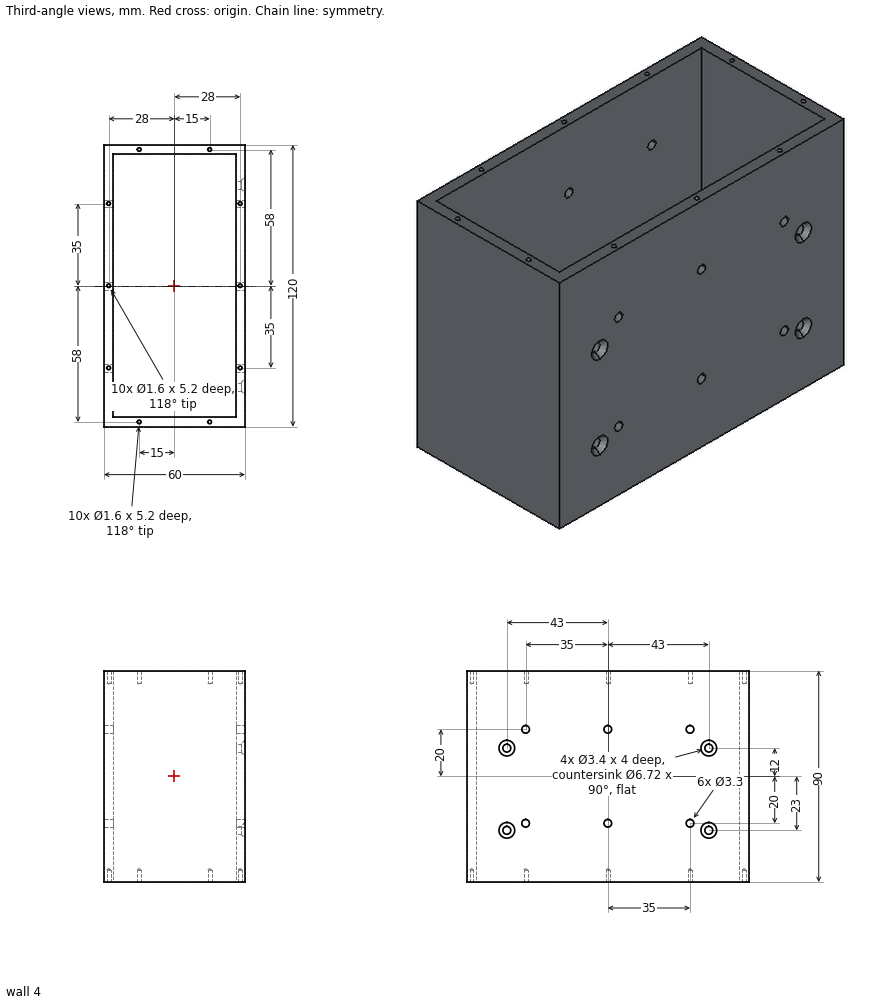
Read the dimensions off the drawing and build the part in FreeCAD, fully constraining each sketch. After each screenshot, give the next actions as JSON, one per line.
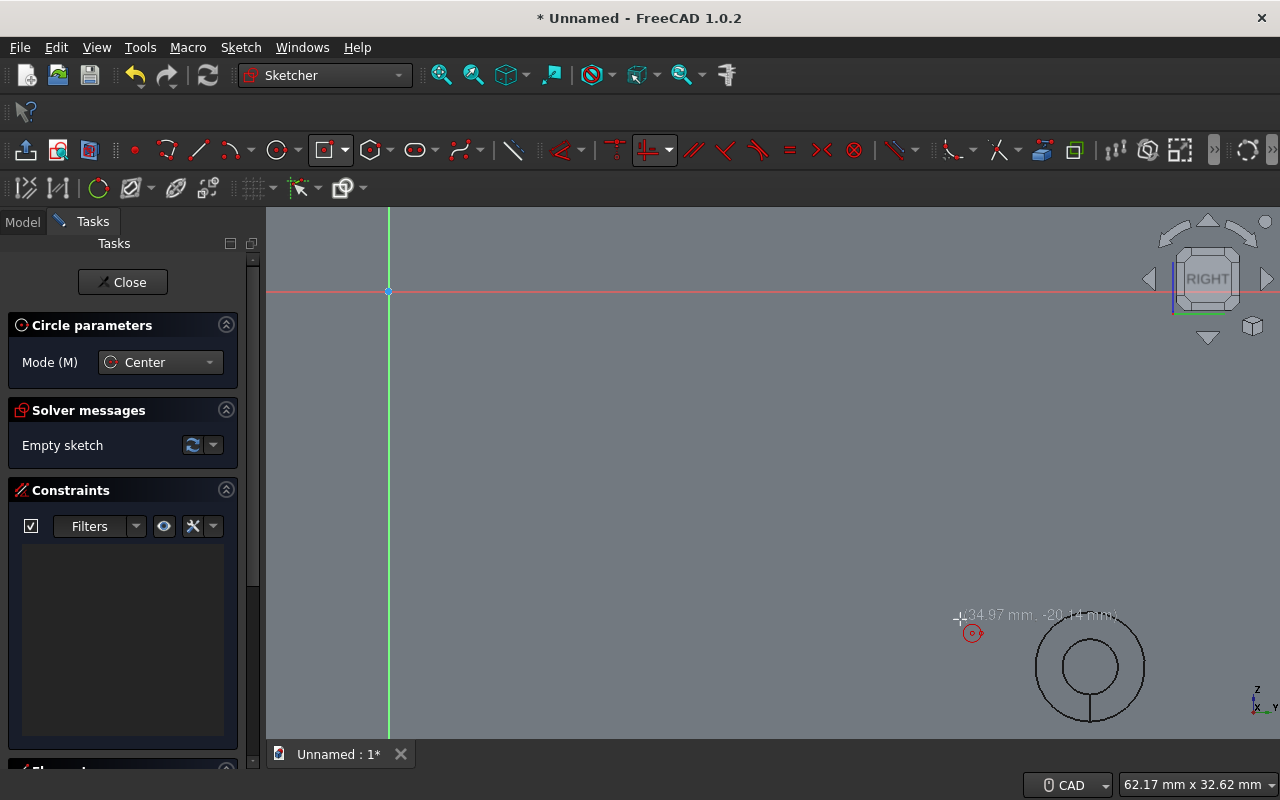
{"action": "left_click", "coordinate": [960, 618]}
{"action": "mouse_move", "coordinate": [979, 599]}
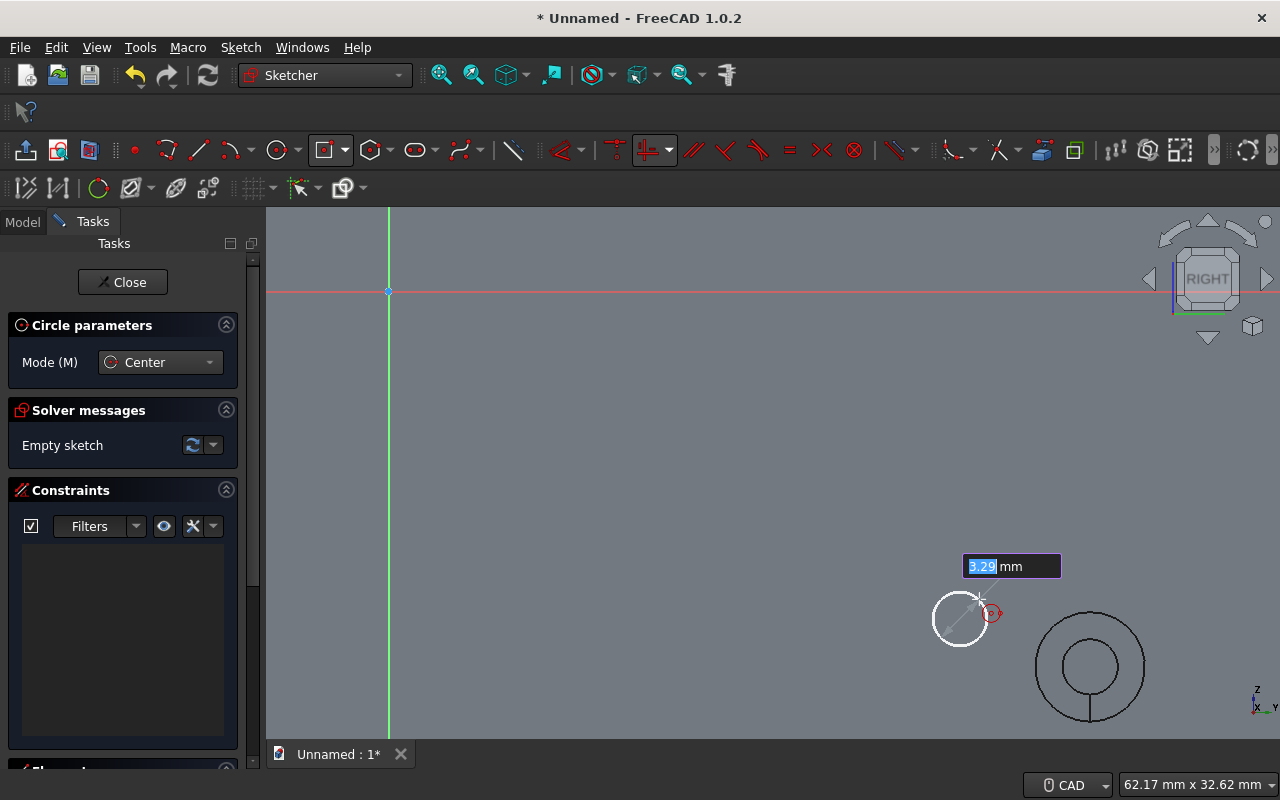
{"action": "type", "text": "3.3"}
{"action": "key", "text": "Return"}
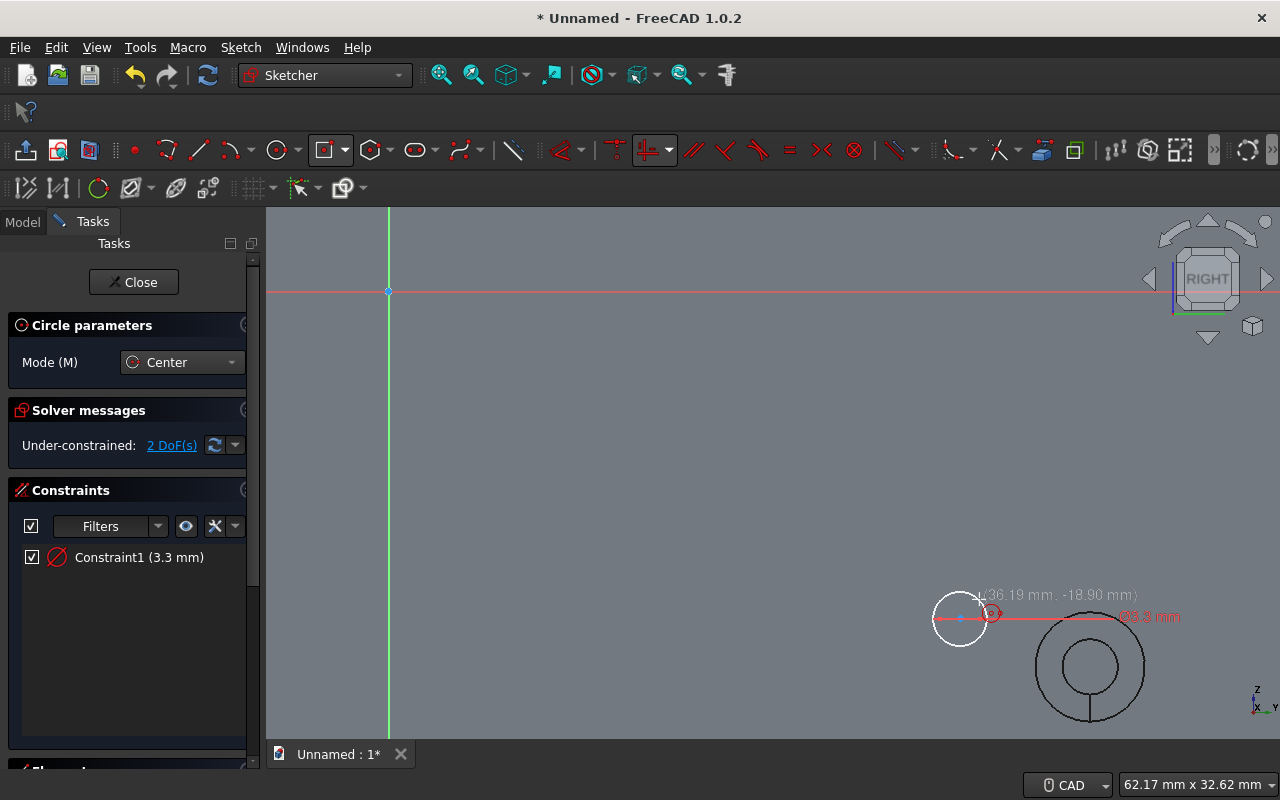
{"action": "scroll", "coordinate": [962, 621], "scroll_direction": "down", "scroll_amount": 4}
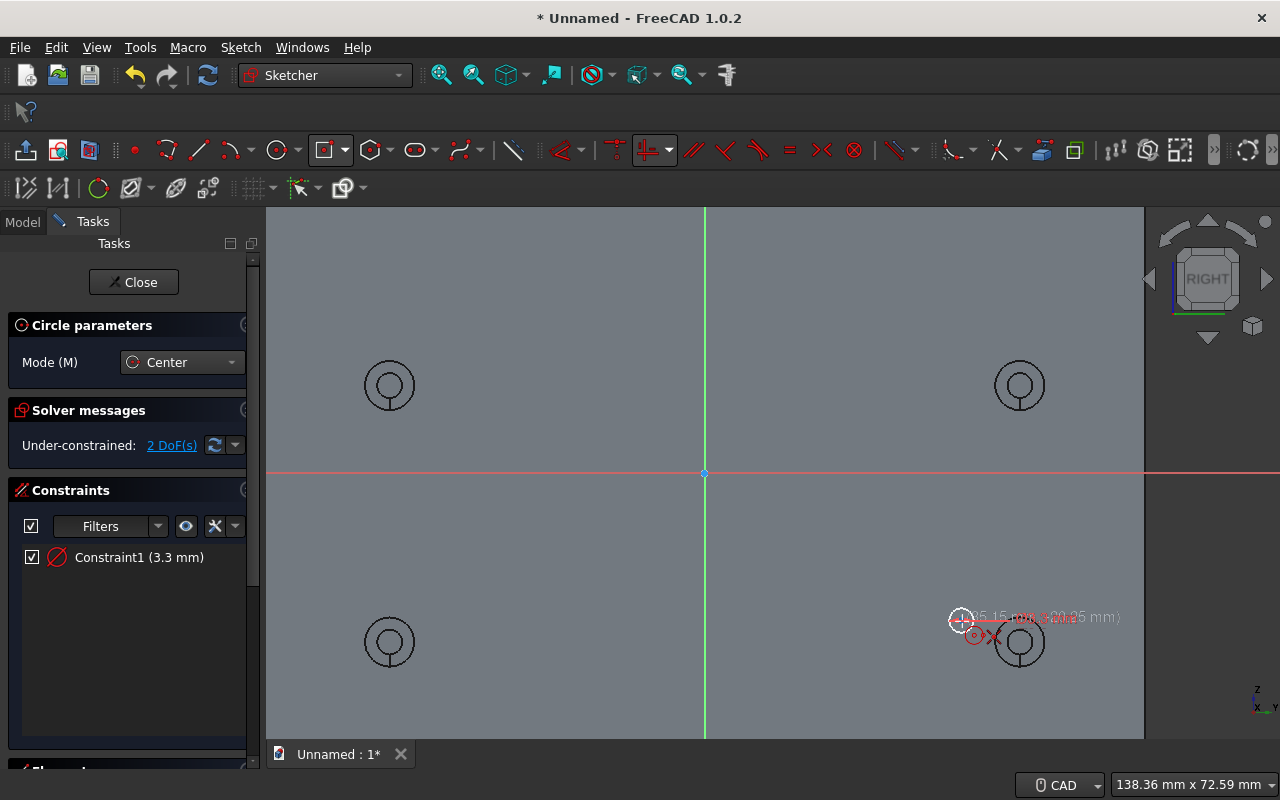
{"action": "scroll", "coordinate": [448, 327], "scroll_direction": "up", "scroll_amount": 4}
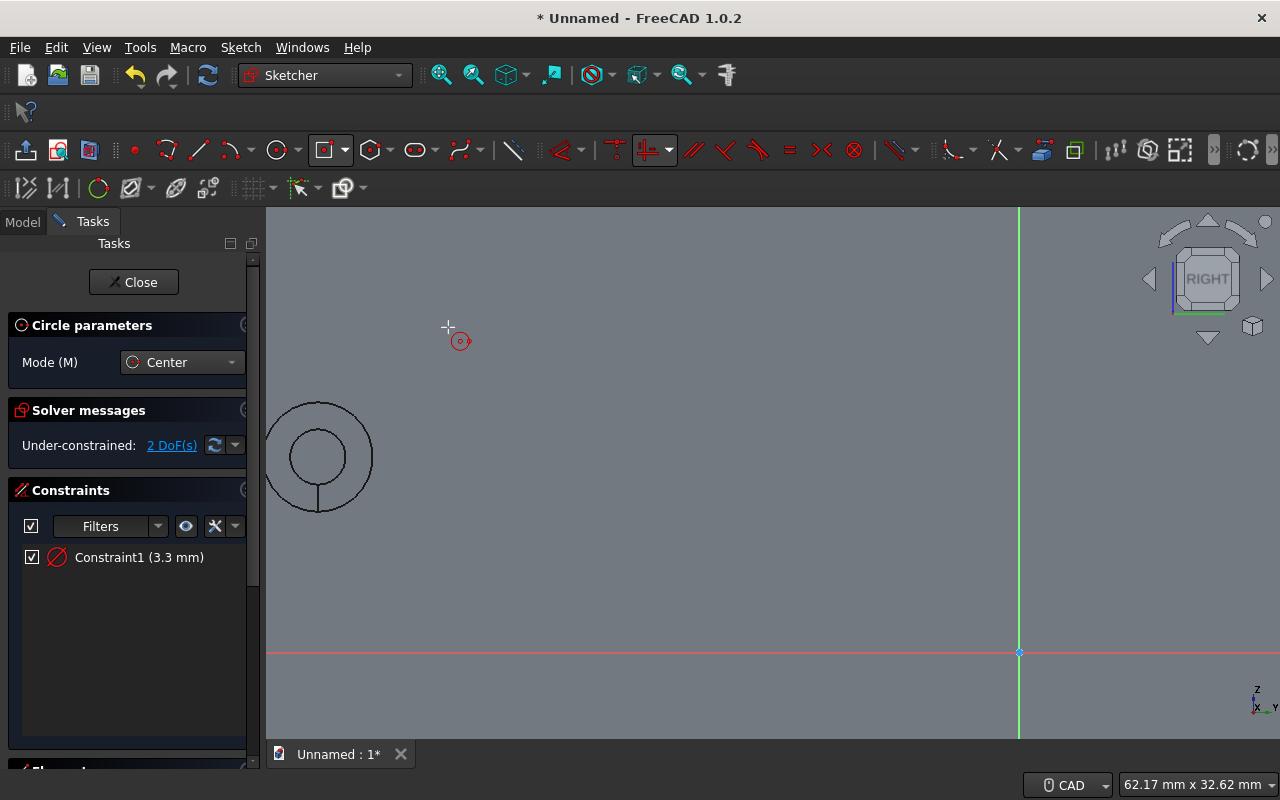
{"action": "left_click", "coordinate": [448, 327]}
{"action": "mouse_move", "coordinate": [467, 308]}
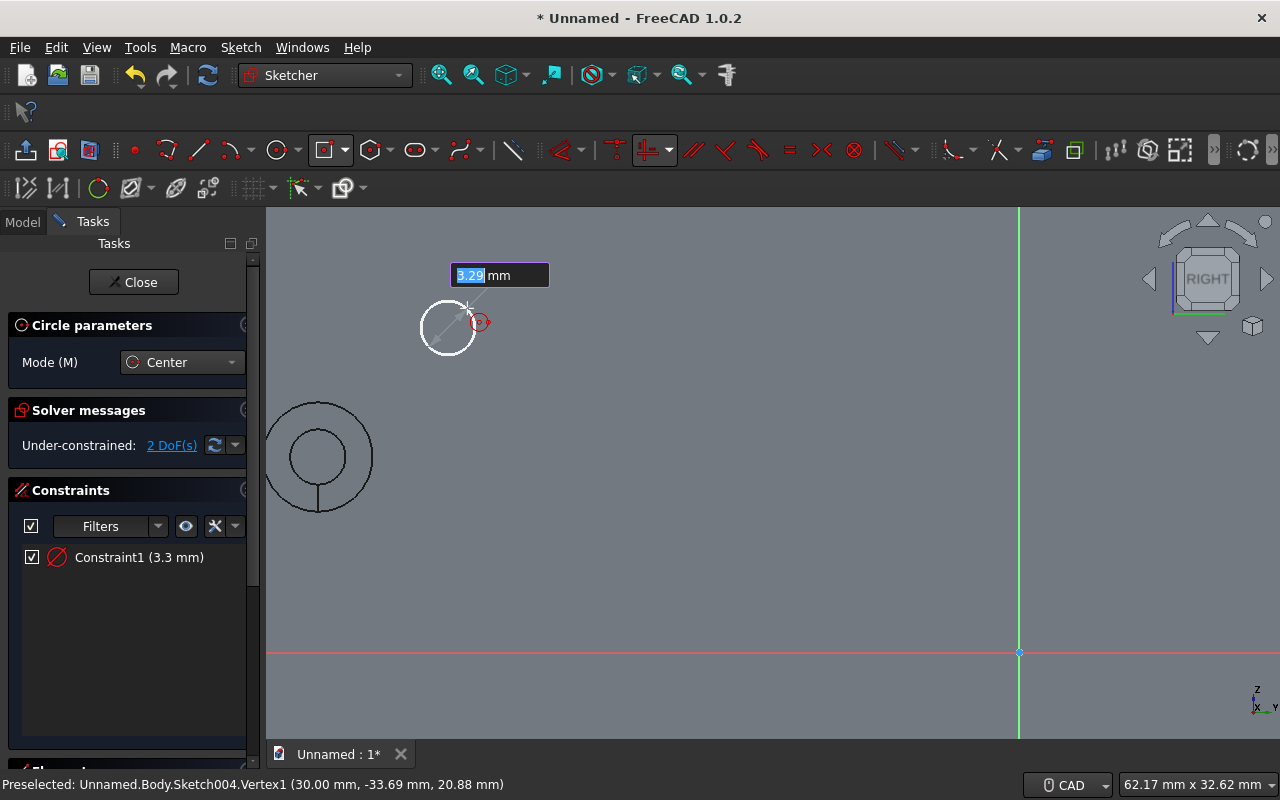
{"action": "type", "text": "3.3"}
{"action": "key", "text": "Return"}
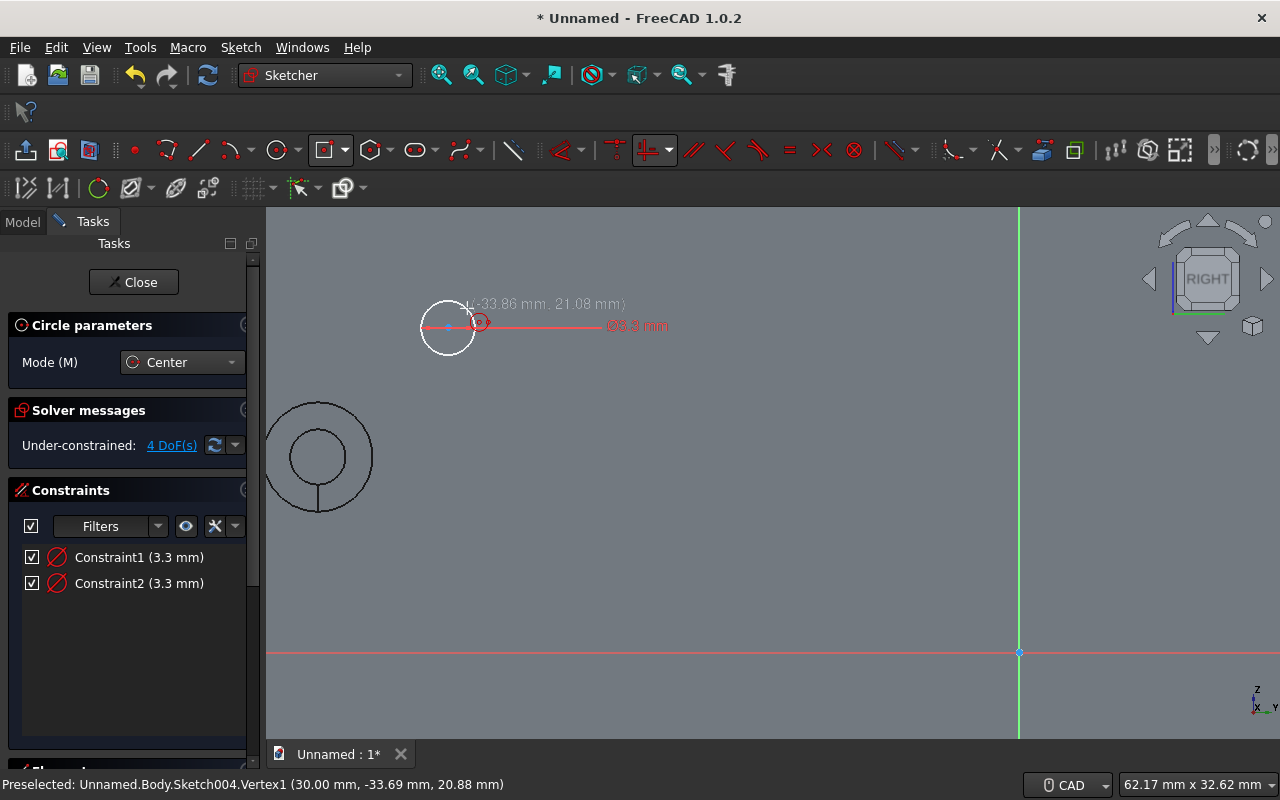
{"action": "scroll", "coordinate": [448, 326], "scroll_direction": "down", "scroll_amount": 4}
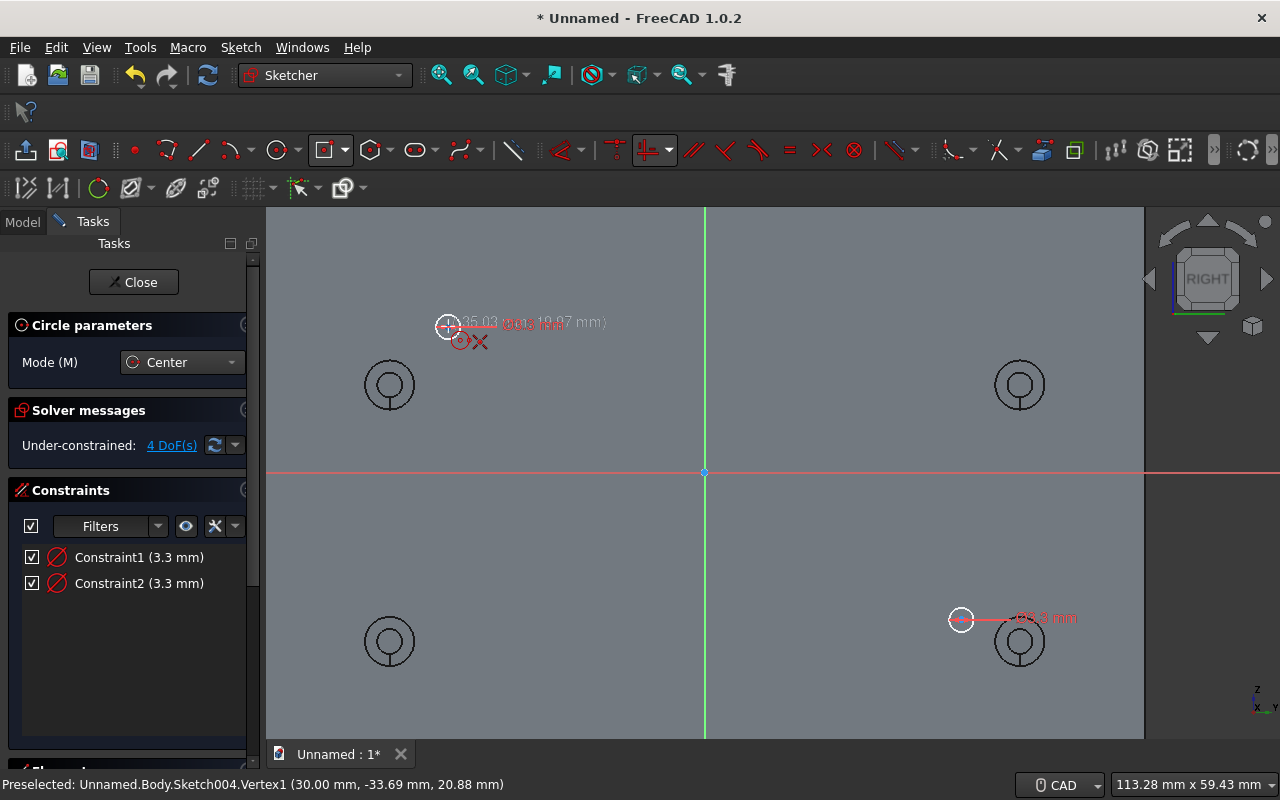
{"action": "scroll", "coordinate": [961, 326], "scroll_direction": "up", "scroll_amount": 4}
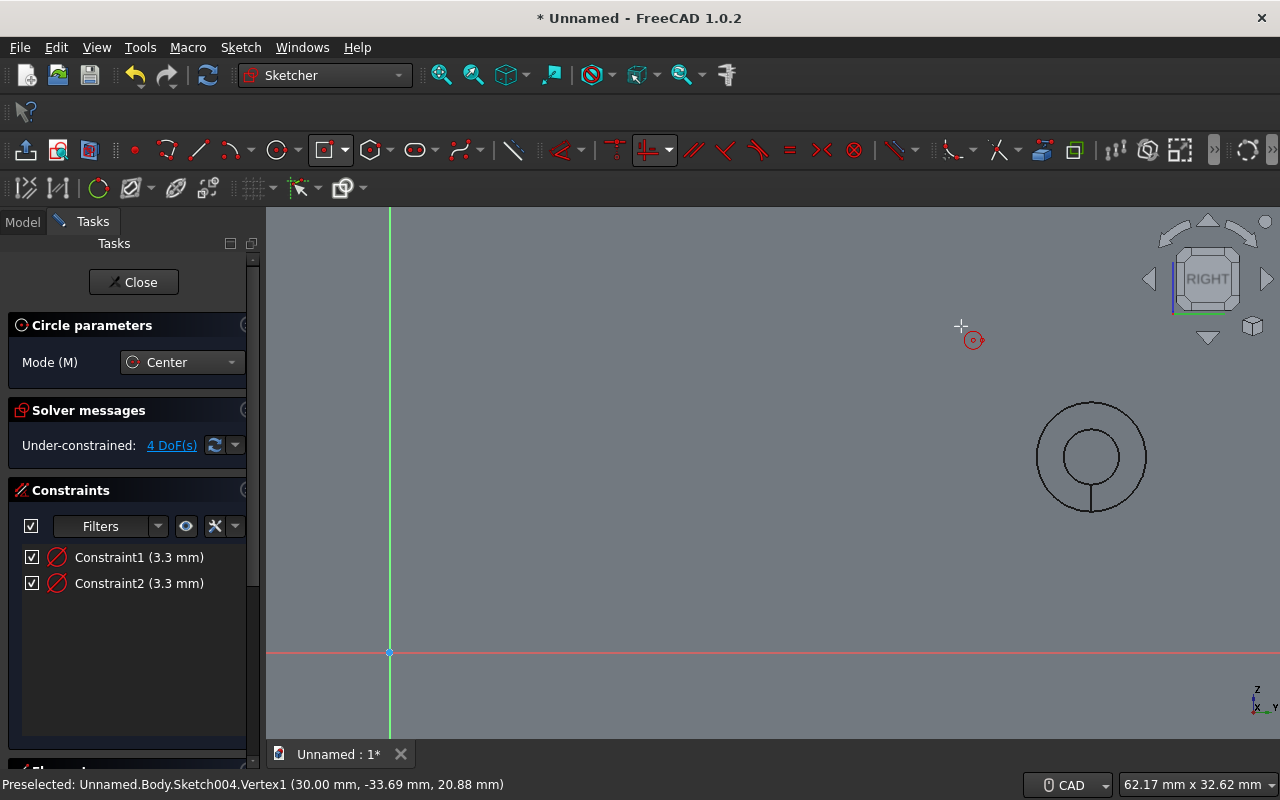
{"action": "left_click", "coordinate": [961, 327]}
{"action": "mouse_move", "coordinate": [980, 308]}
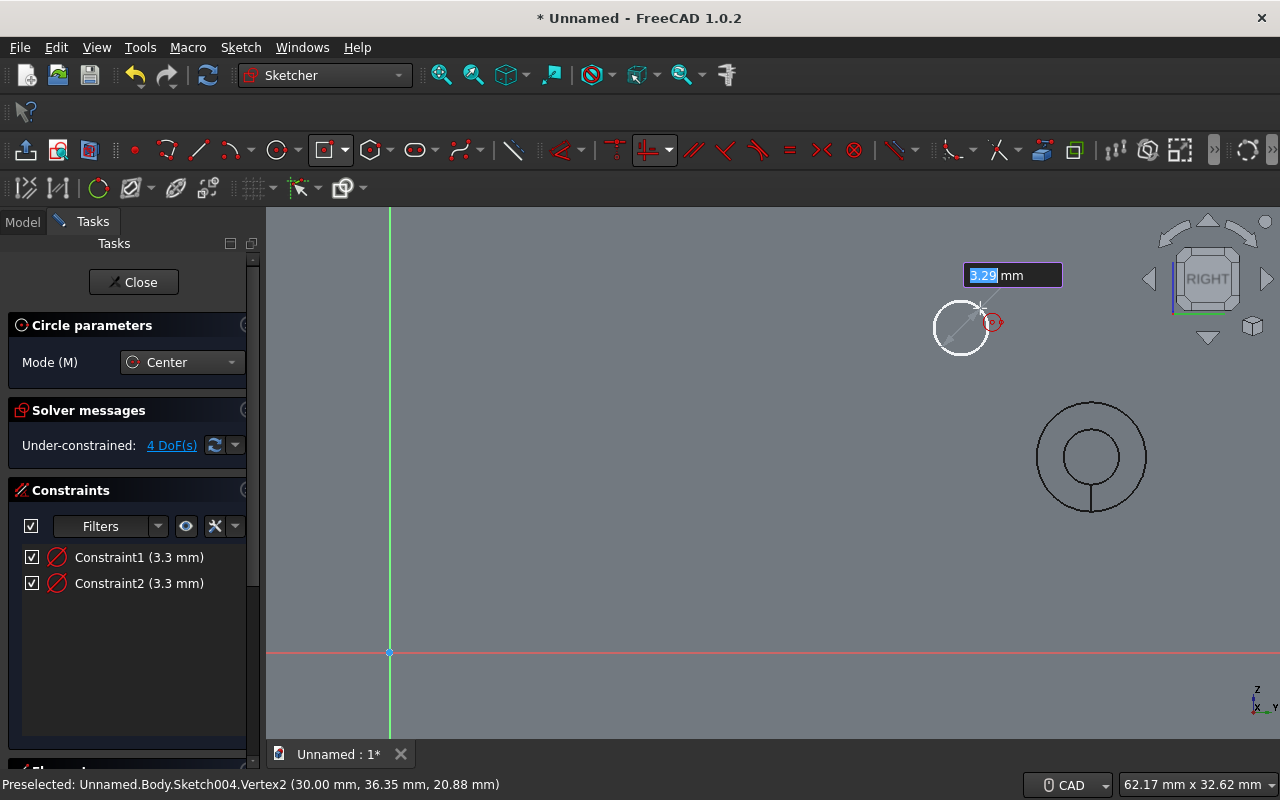
{"action": "type", "text": "3.3"}
{"action": "key", "text": "Return"}